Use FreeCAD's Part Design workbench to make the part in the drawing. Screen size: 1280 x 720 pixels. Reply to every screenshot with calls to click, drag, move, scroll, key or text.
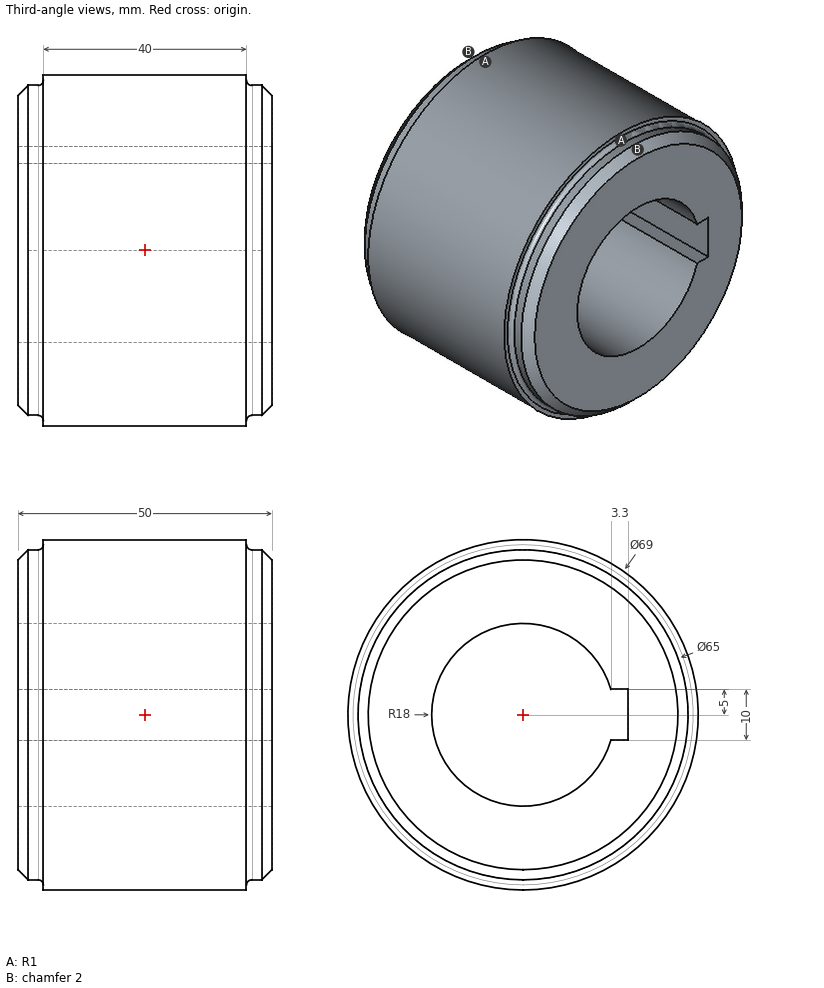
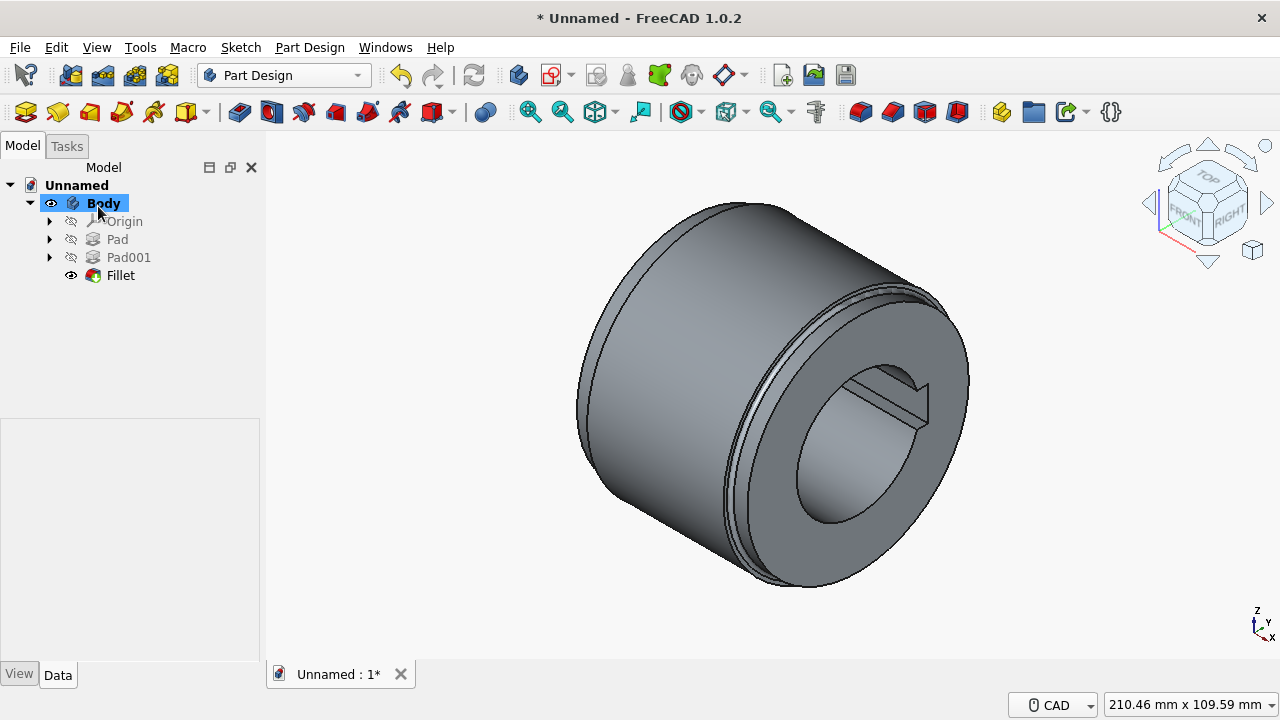
click(747, 507)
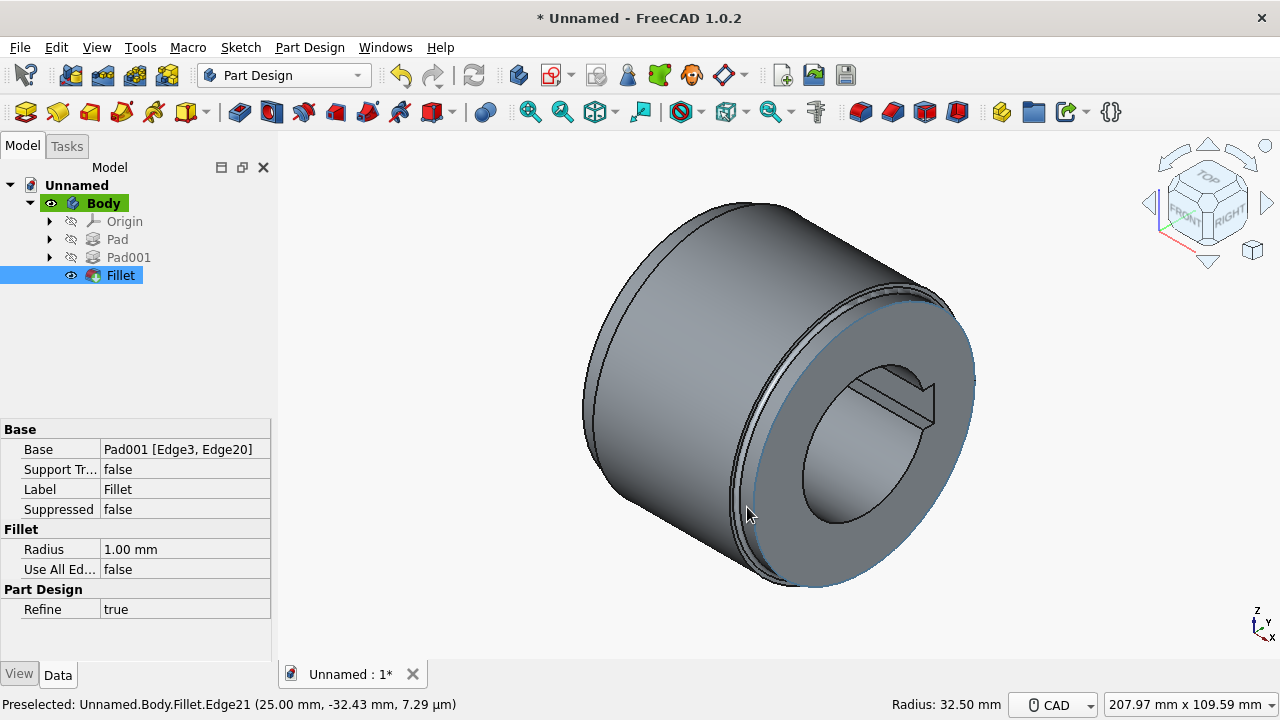
key(2)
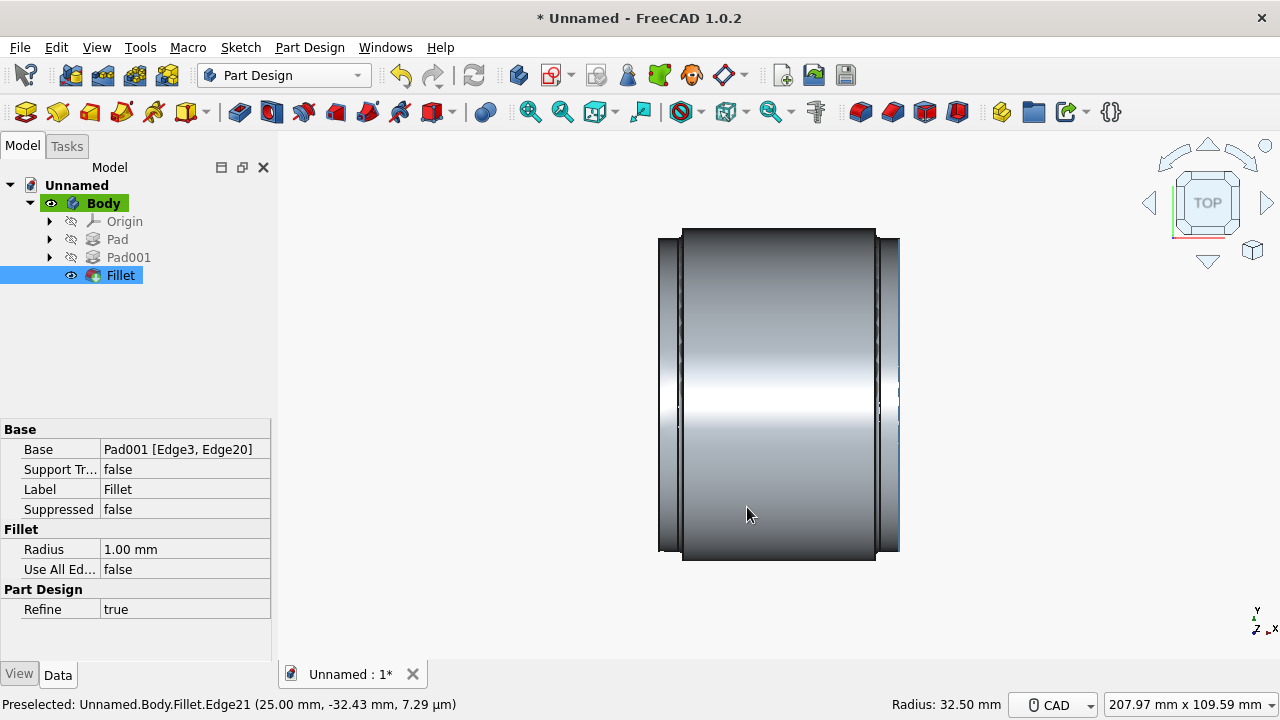
click(659, 346, ctrl)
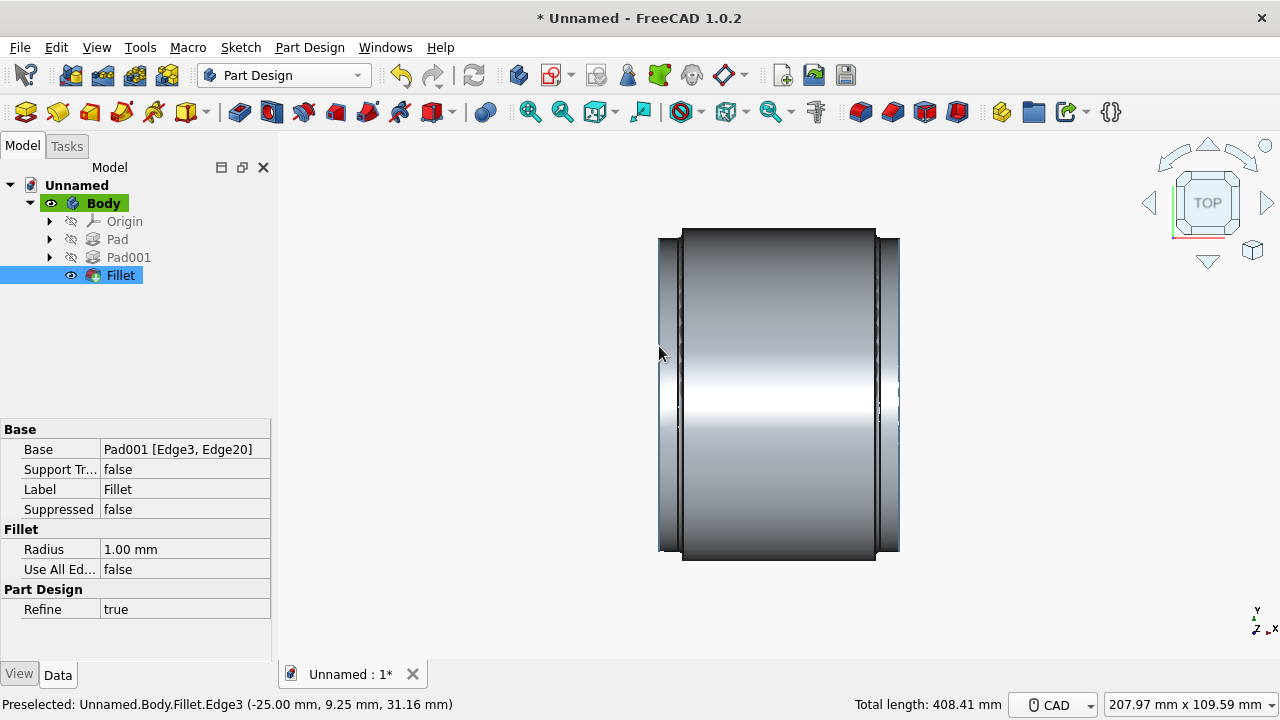
click(894, 112)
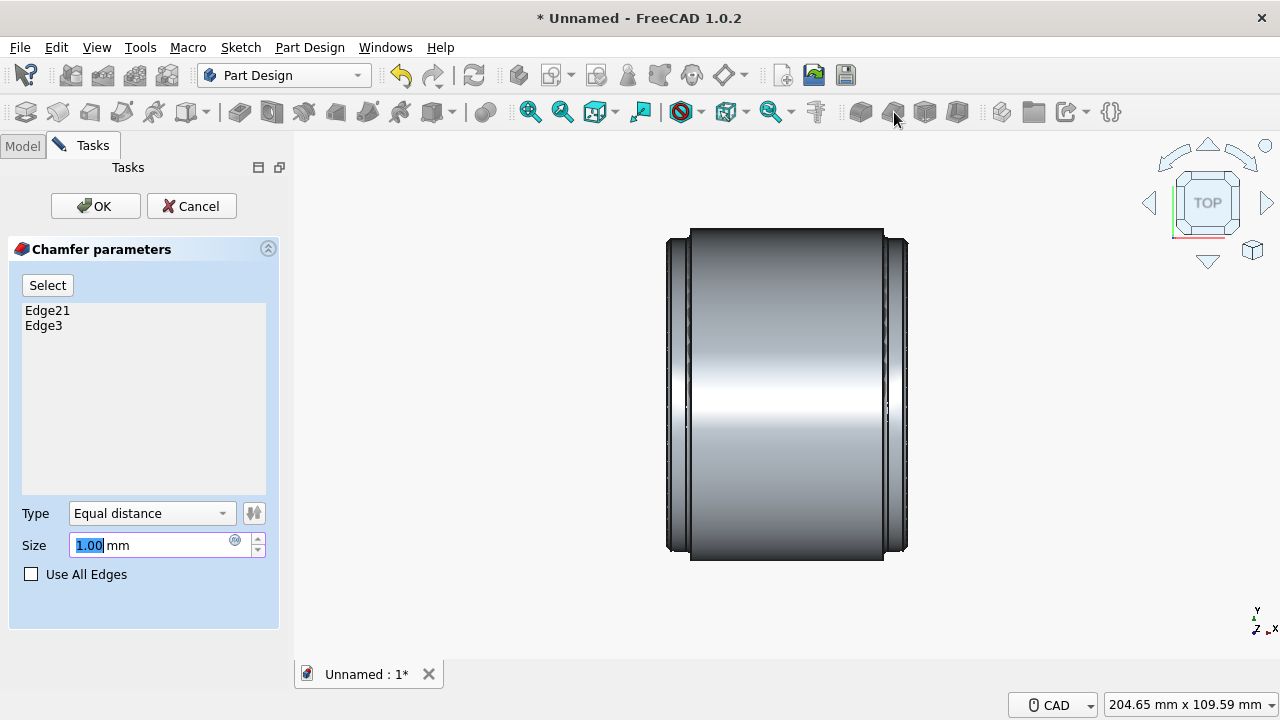
text(2)
key(Tab)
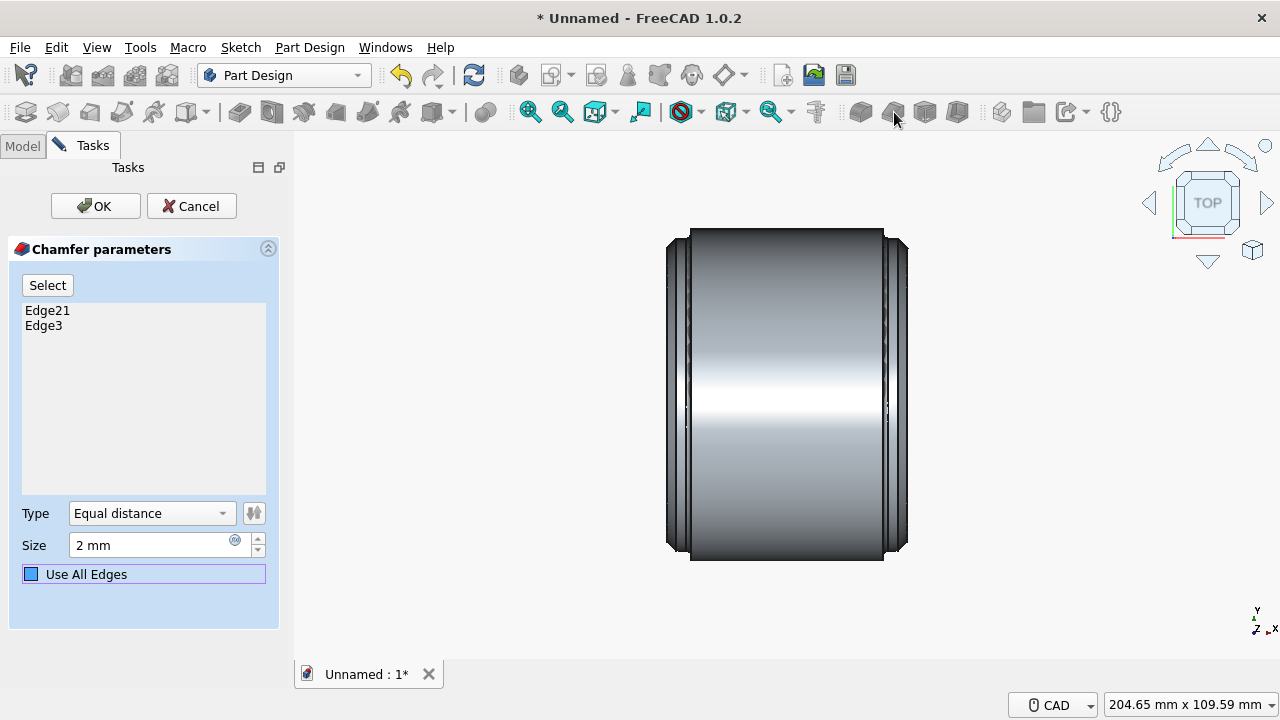
click(96, 206)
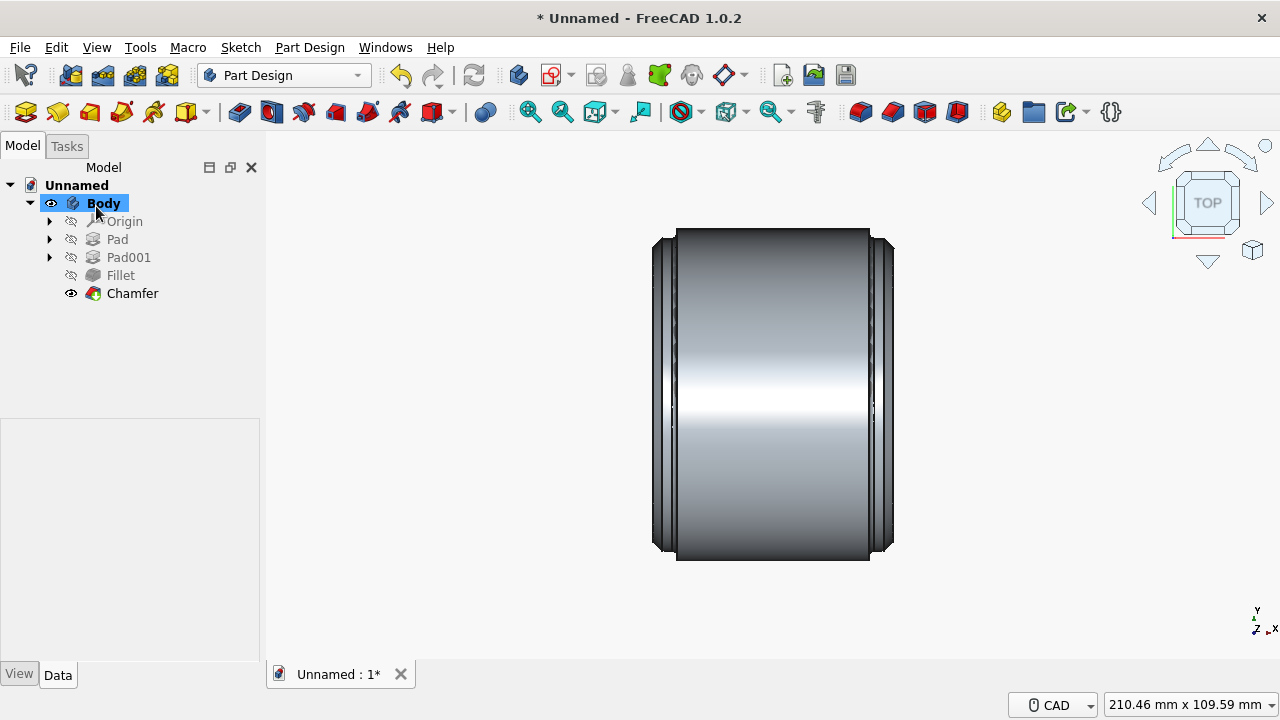
key(0)